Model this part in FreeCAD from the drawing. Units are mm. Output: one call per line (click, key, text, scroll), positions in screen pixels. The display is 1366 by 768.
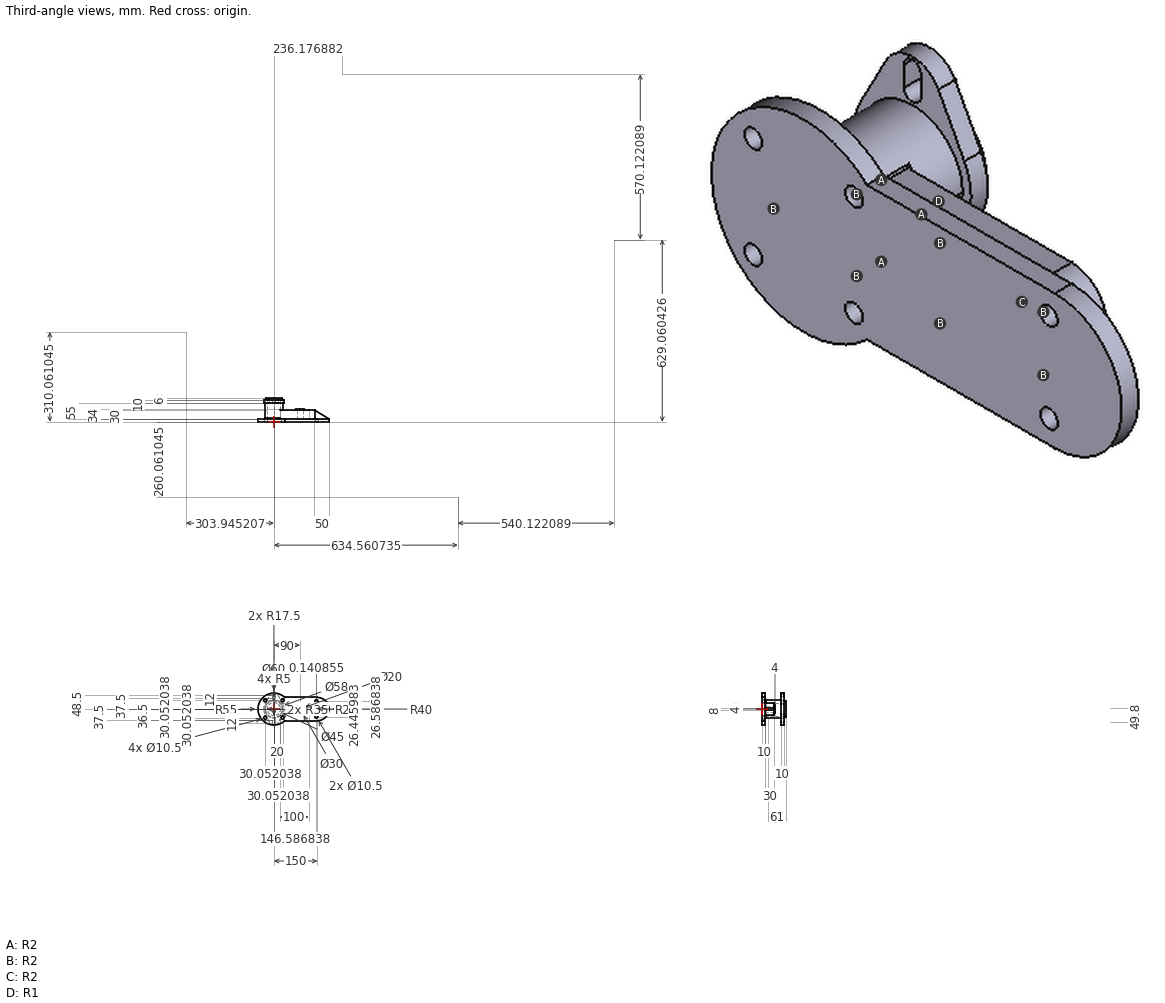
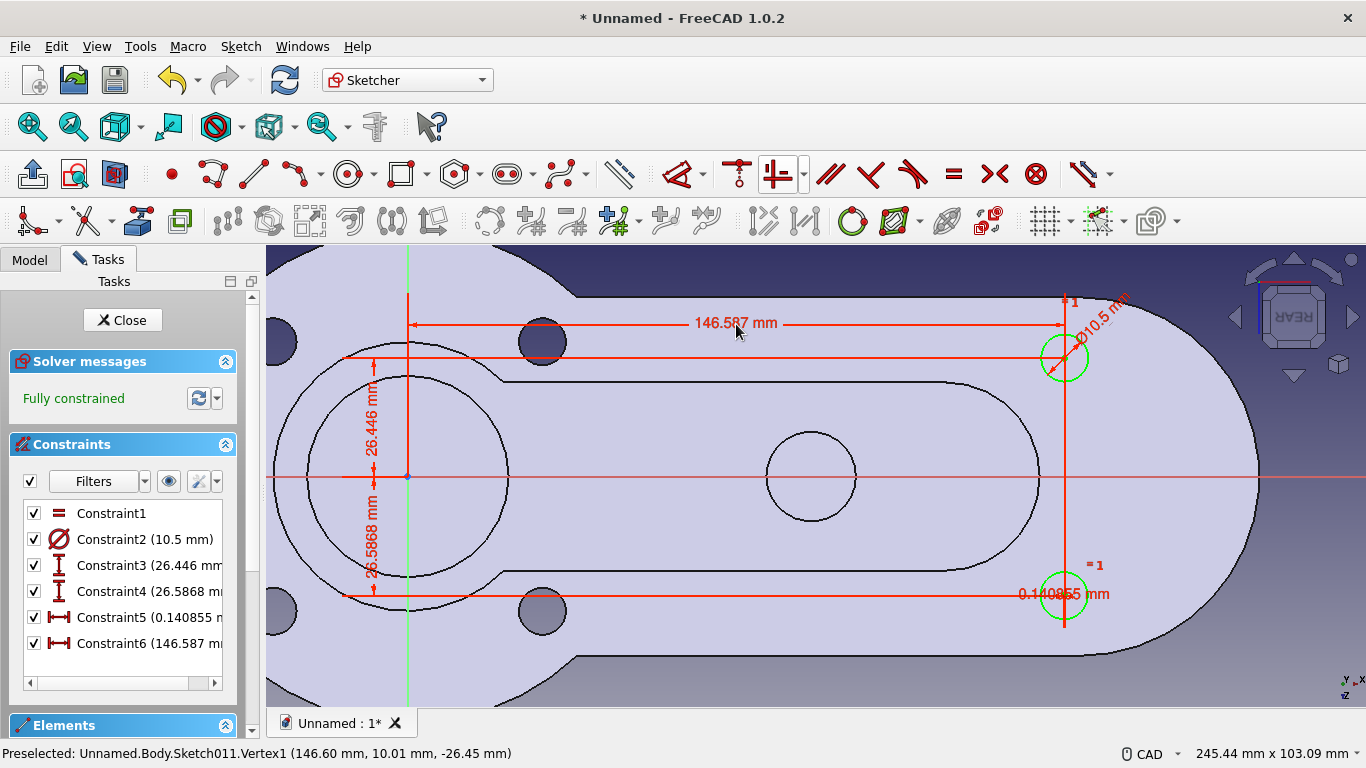
click(123, 320)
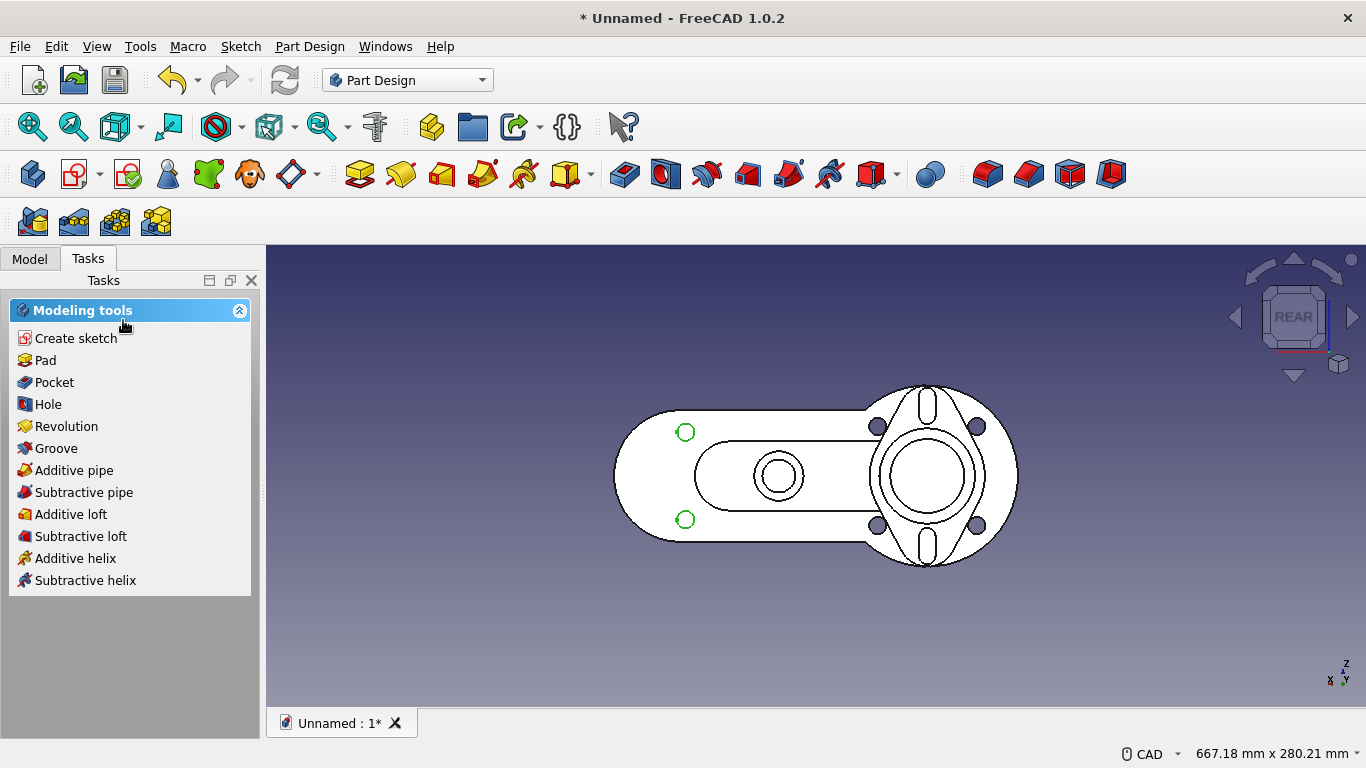
click(625, 174)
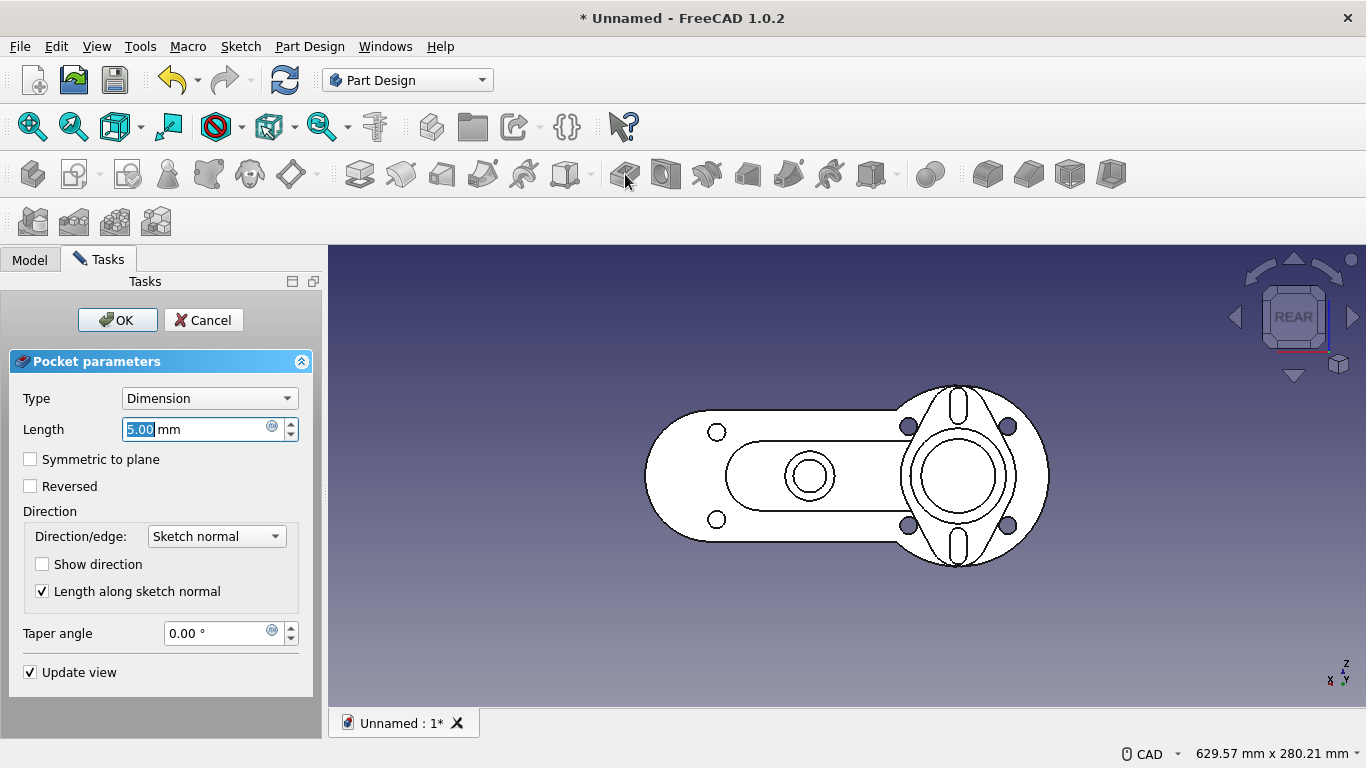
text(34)
key(Tab)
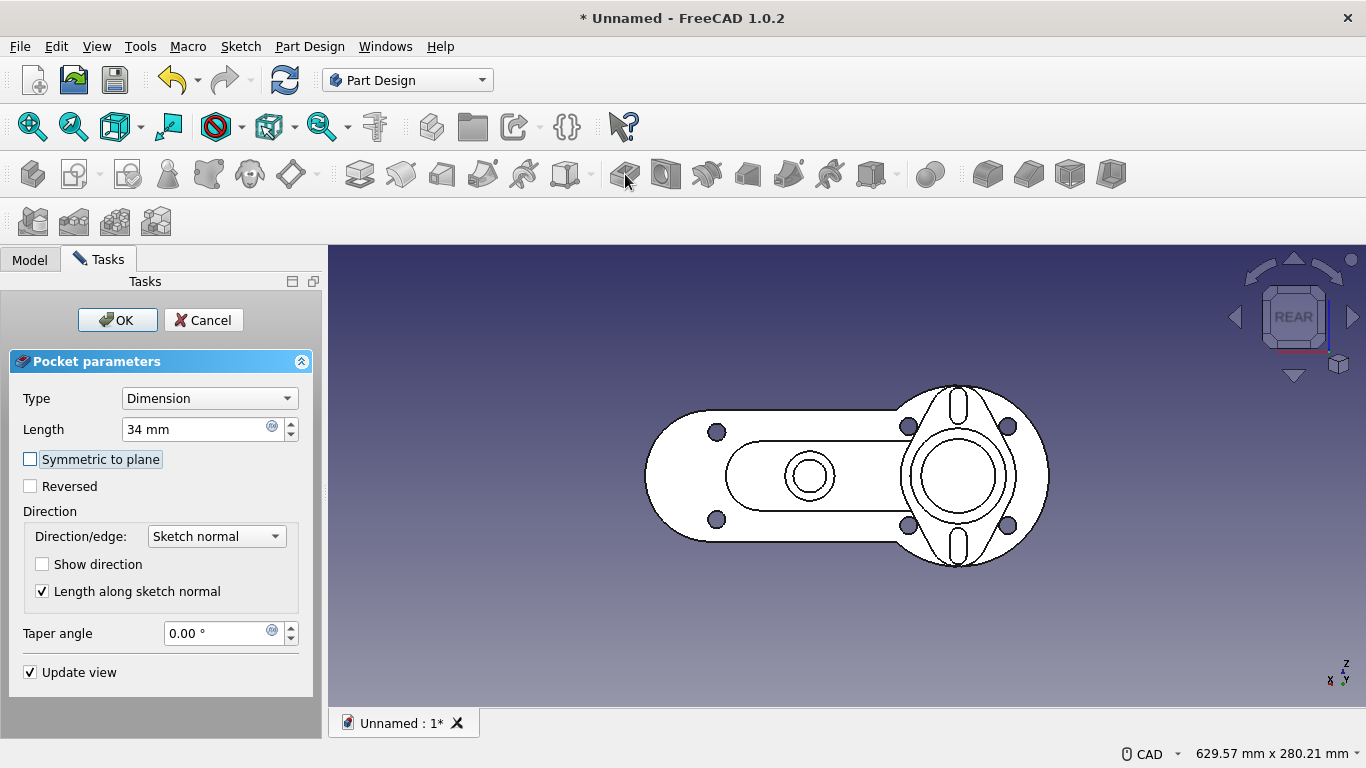
click(118, 320)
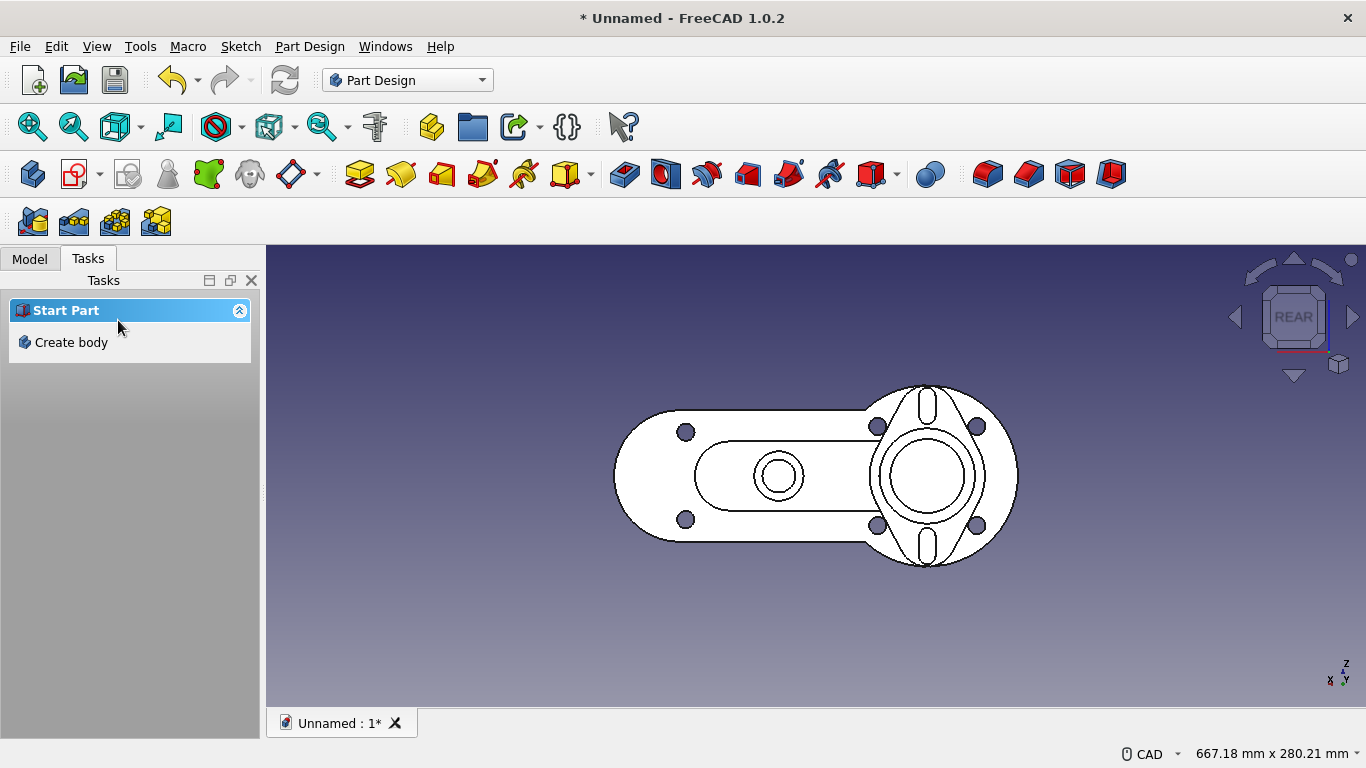
click(33, 128)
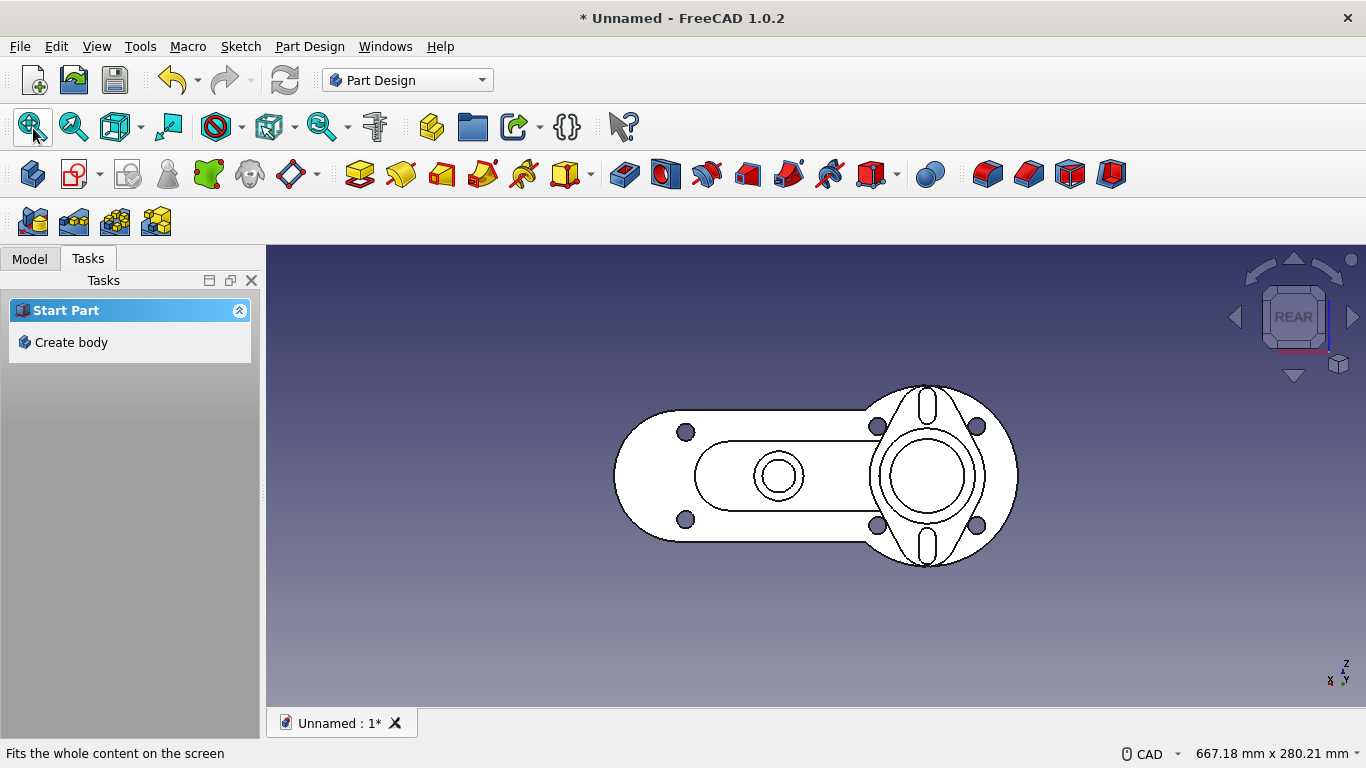
click(30, 258)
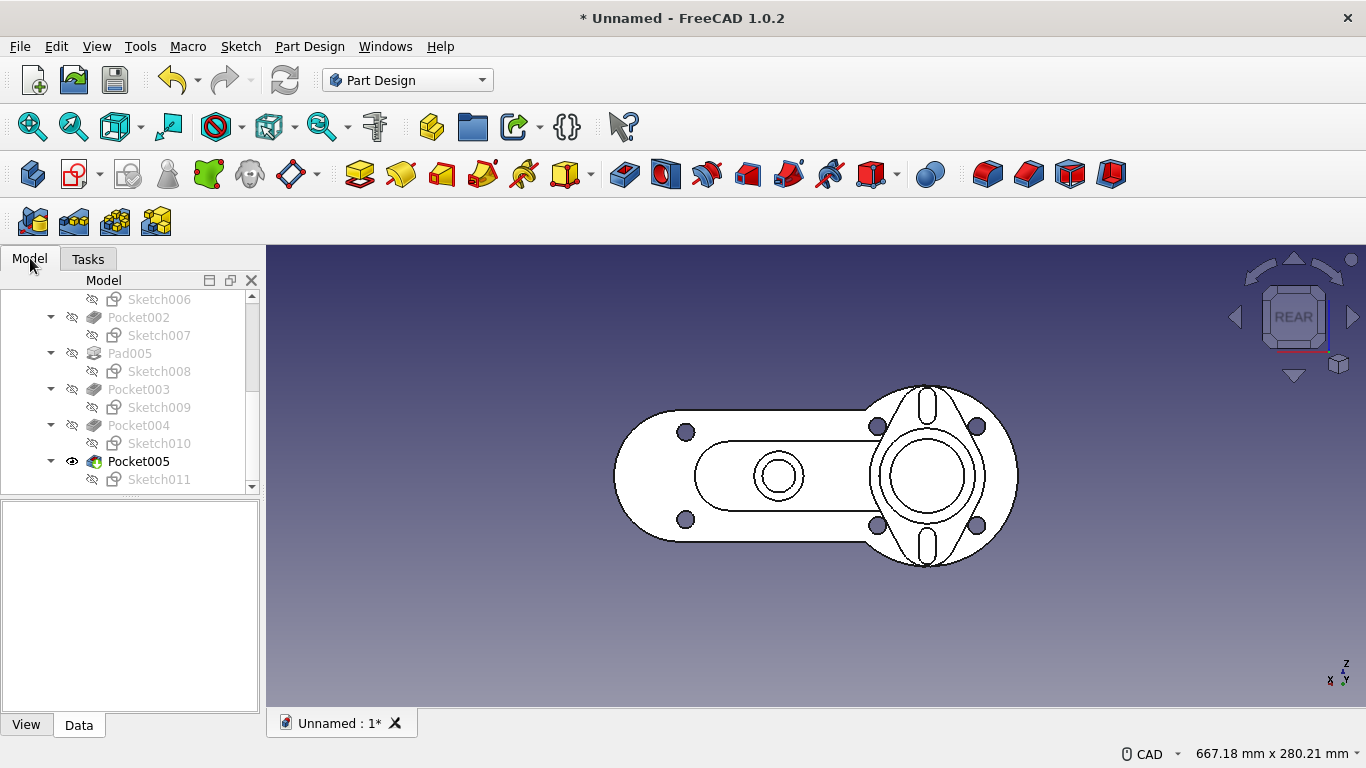
scroll(161, 385, down, 3)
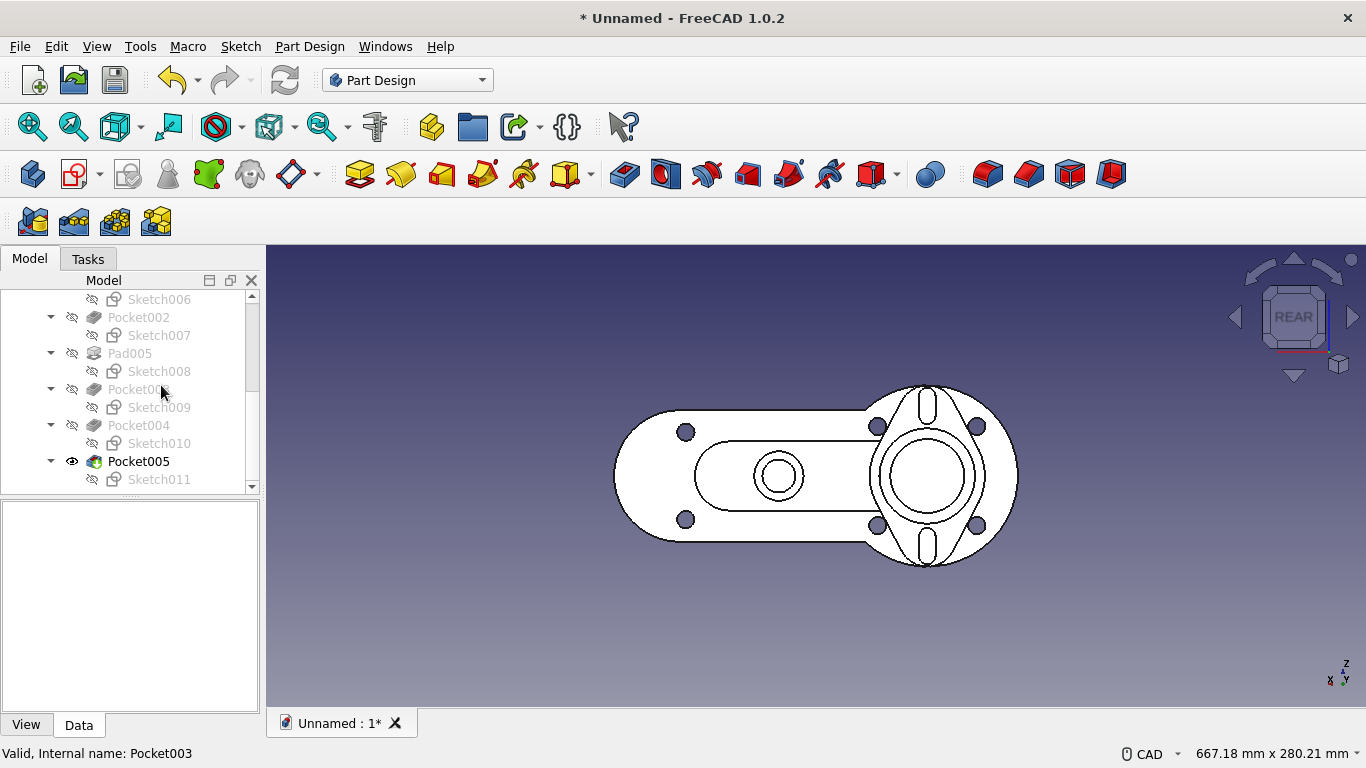
scroll(161, 385, up, 15)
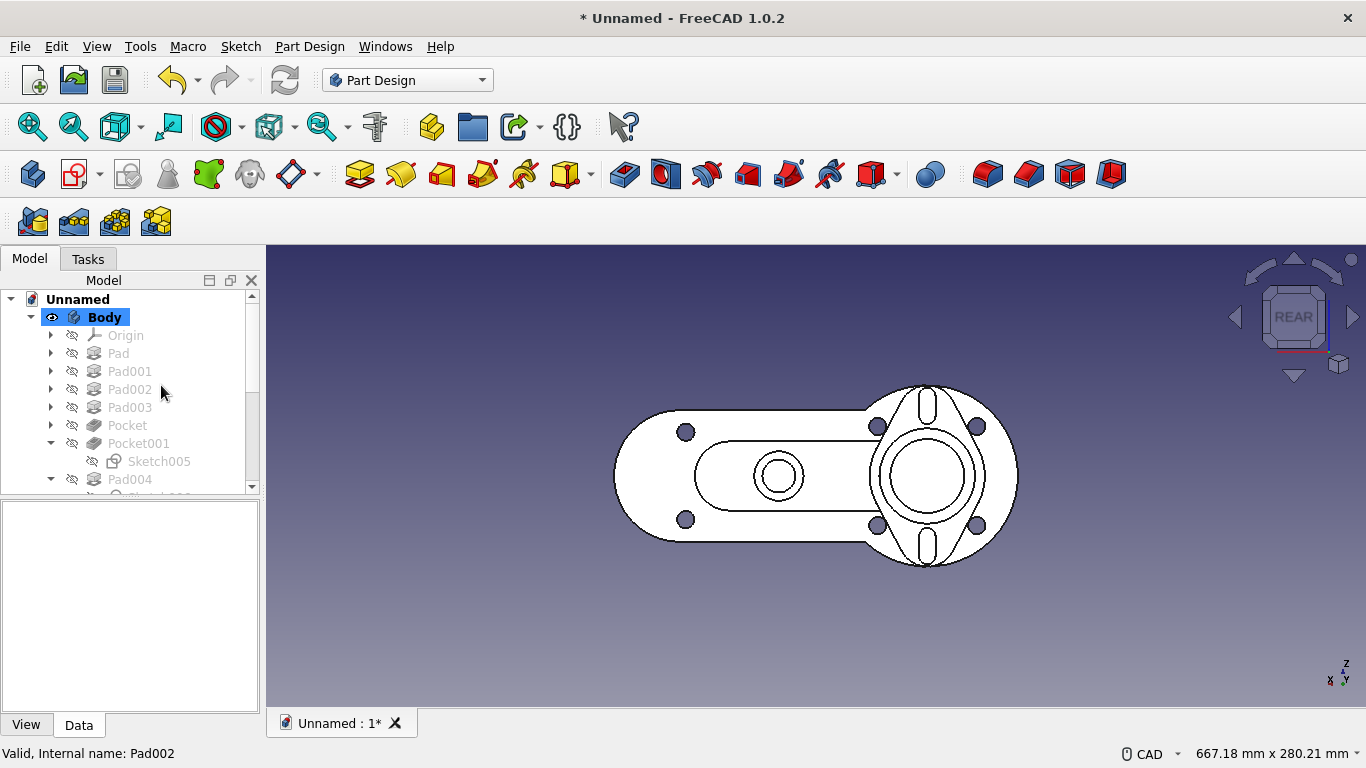
click(51, 335)